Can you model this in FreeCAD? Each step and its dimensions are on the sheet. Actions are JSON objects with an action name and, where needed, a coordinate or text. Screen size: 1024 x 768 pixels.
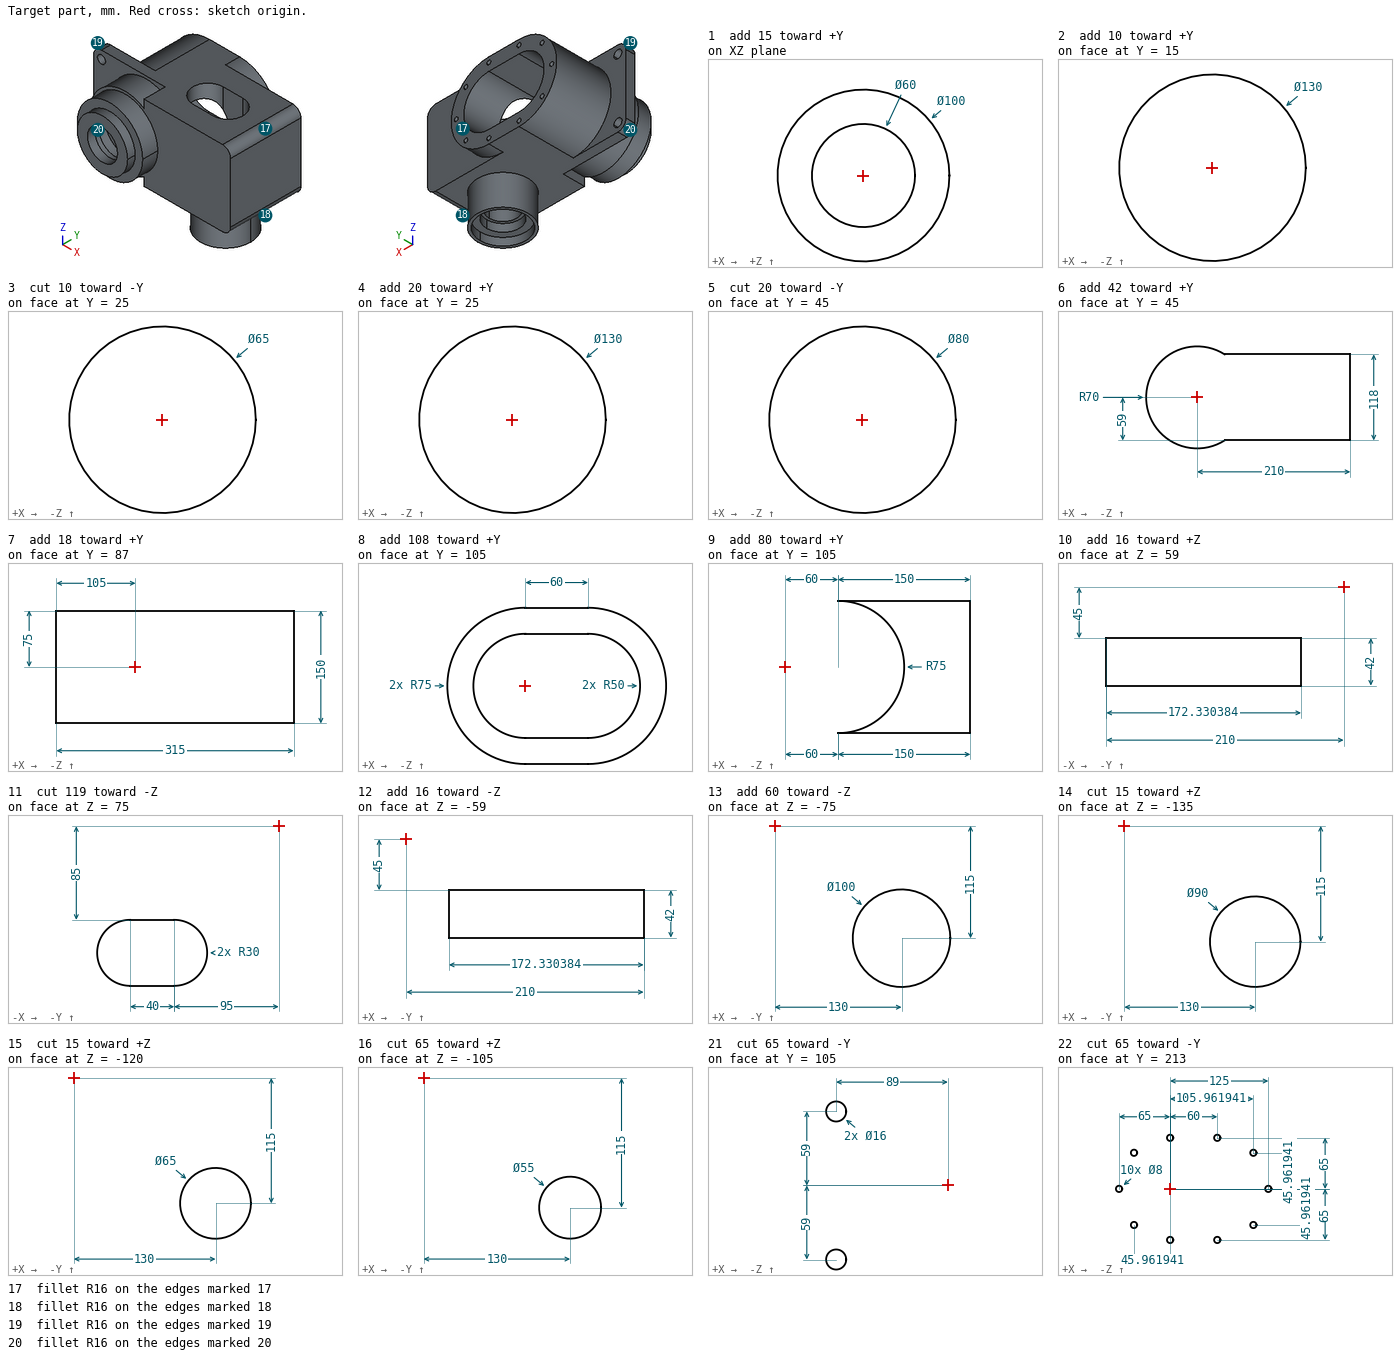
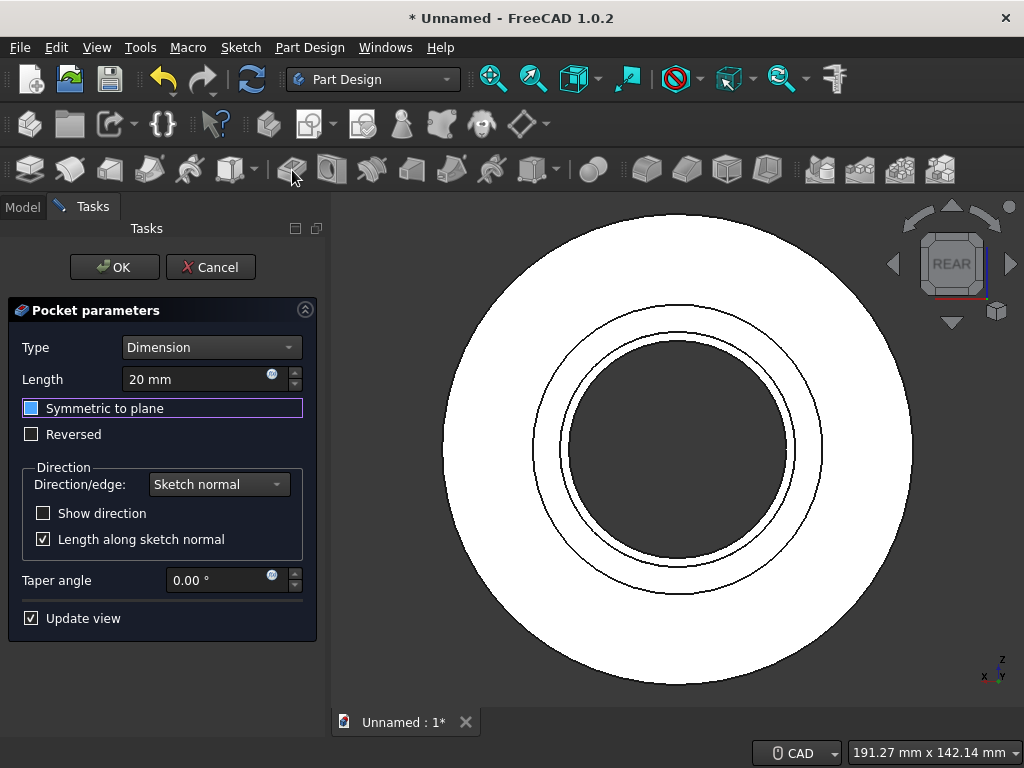
{"action": "left_click", "coordinate": [115, 267]}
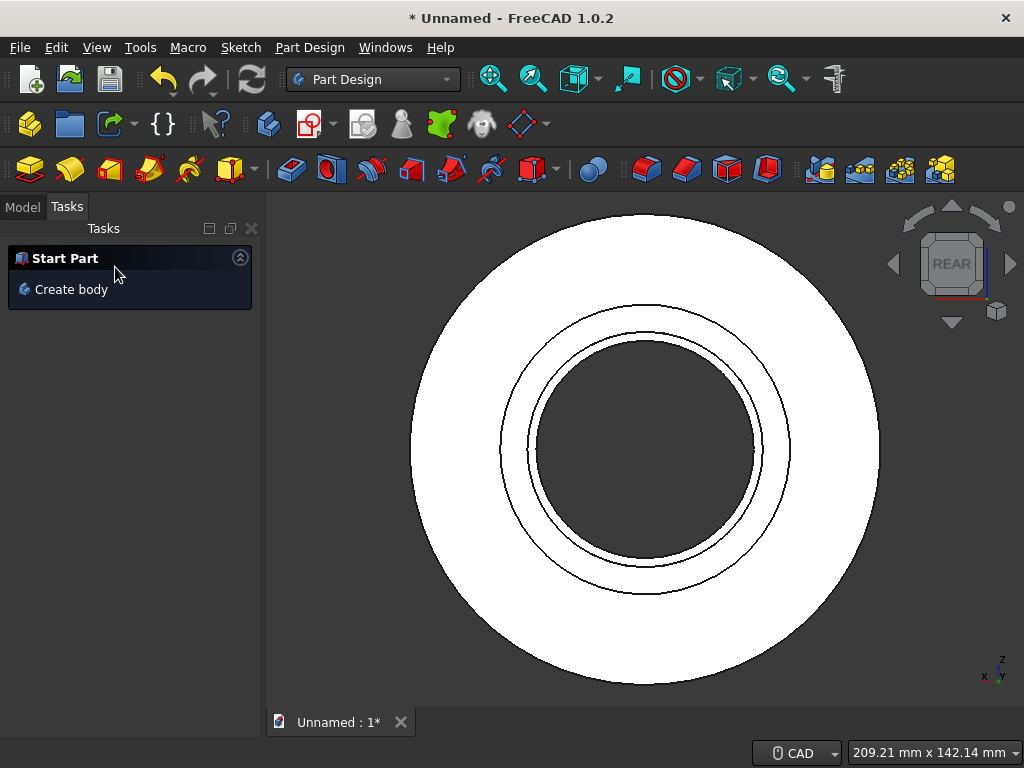
{"action": "left_click", "coordinate": [511, 583]}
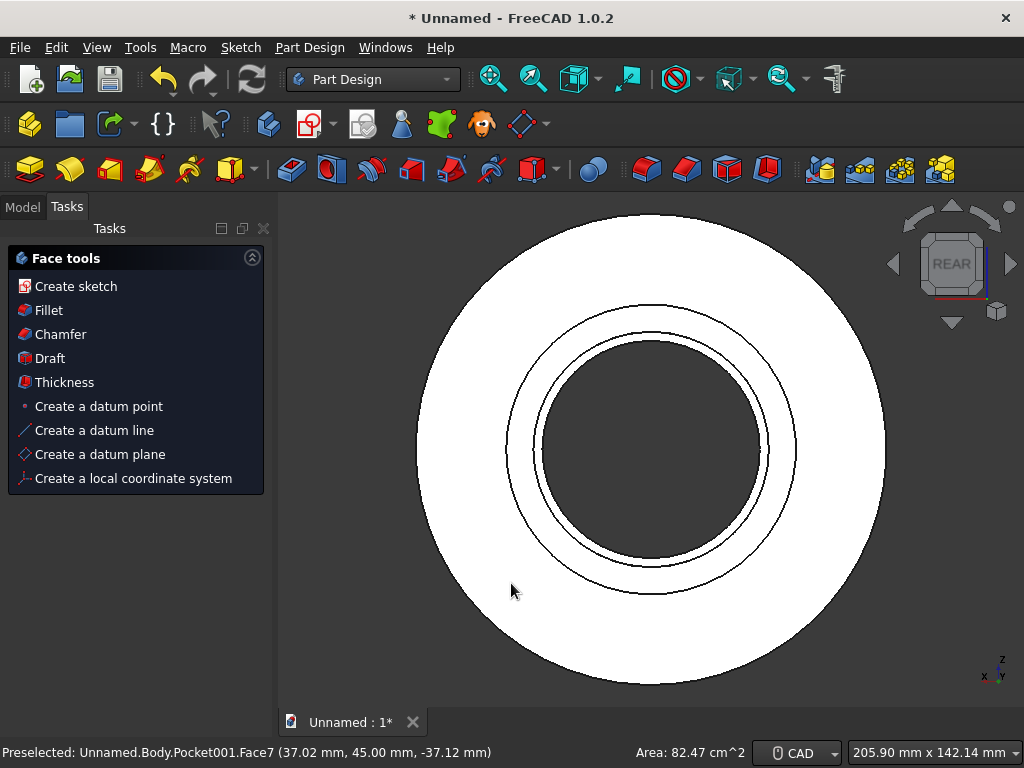
{"action": "left_click", "coordinate": [310, 124]}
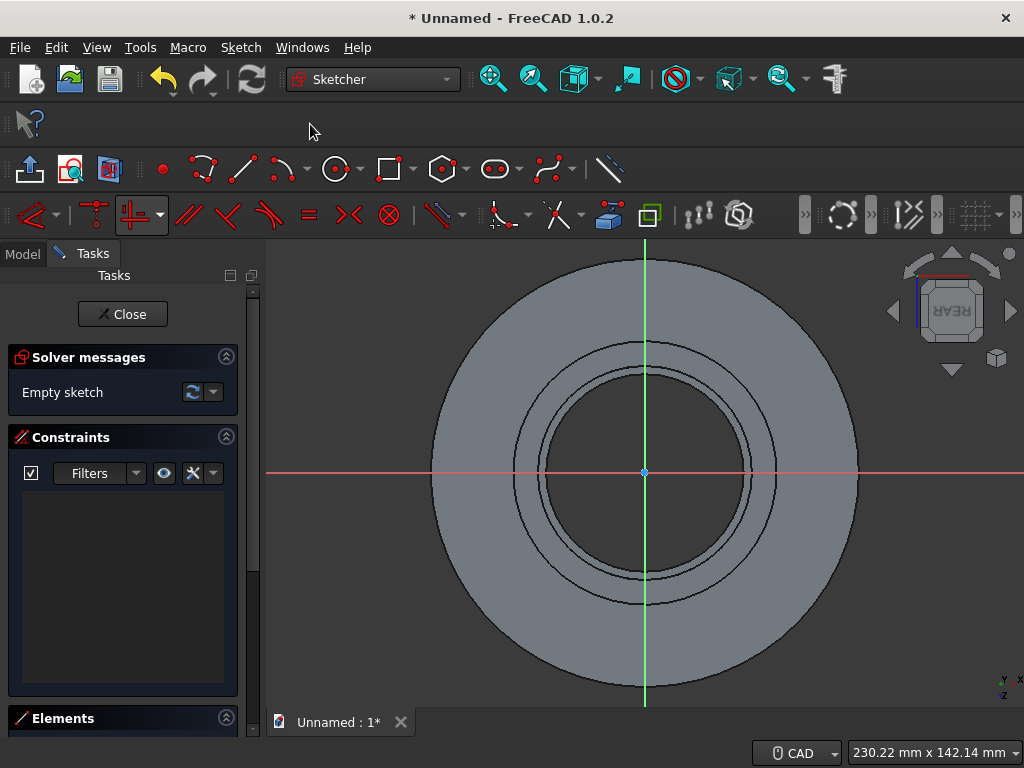
{"action": "scroll", "coordinate": [333, 473], "scroll_direction": "down", "scroll_amount": 4}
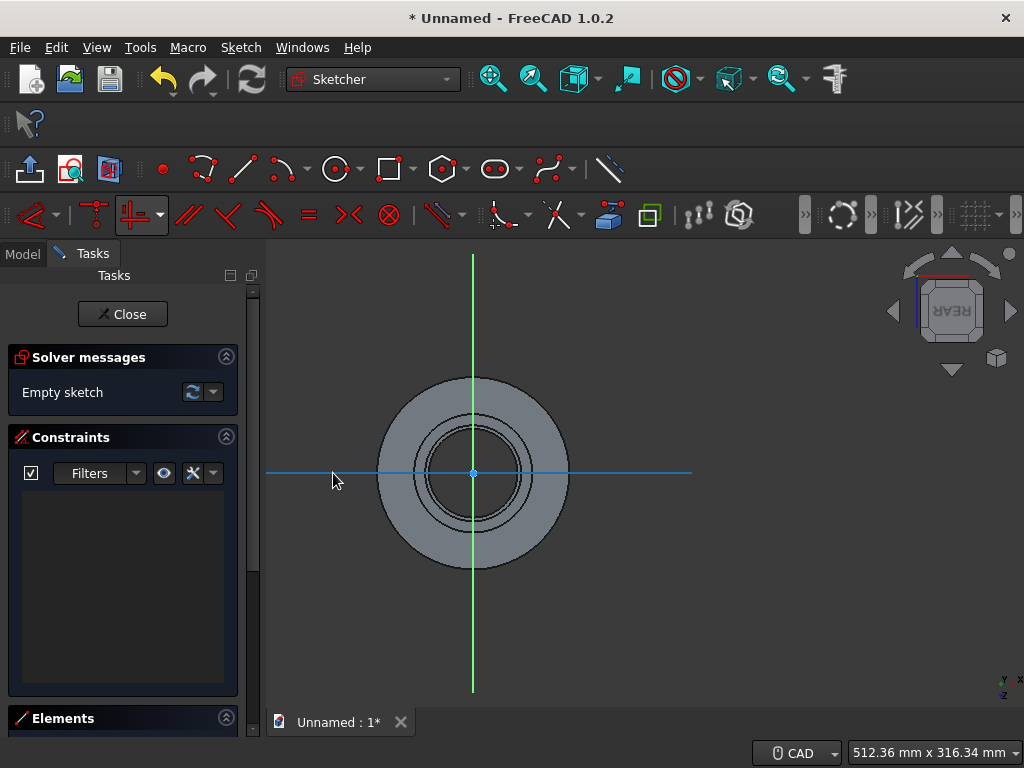
{"action": "left_click", "coordinate": [204, 170]}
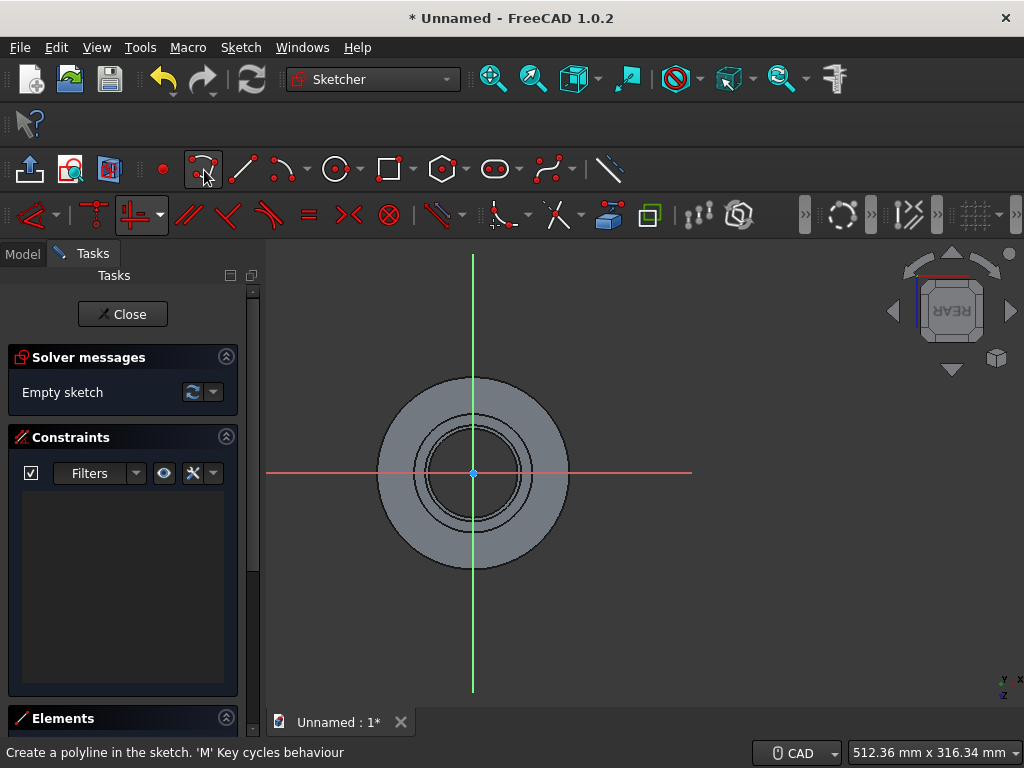
{"action": "left_click", "coordinate": [529, 561]}
{"action": "left_click", "coordinate": [784, 561]}
{"action": "left_click", "coordinate": [784, 386]}
{"action": "left_click", "coordinate": [529, 386]}
{"action": "right_click", "coordinate": [529, 386]}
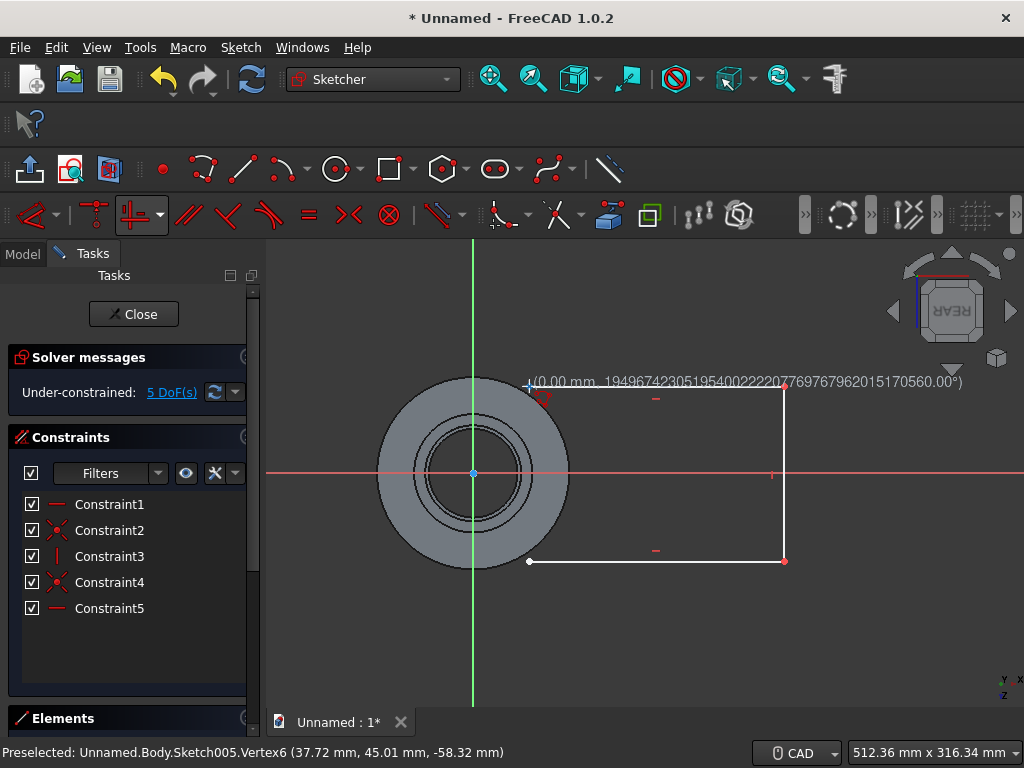
{"action": "key", "text": "g 3 a"}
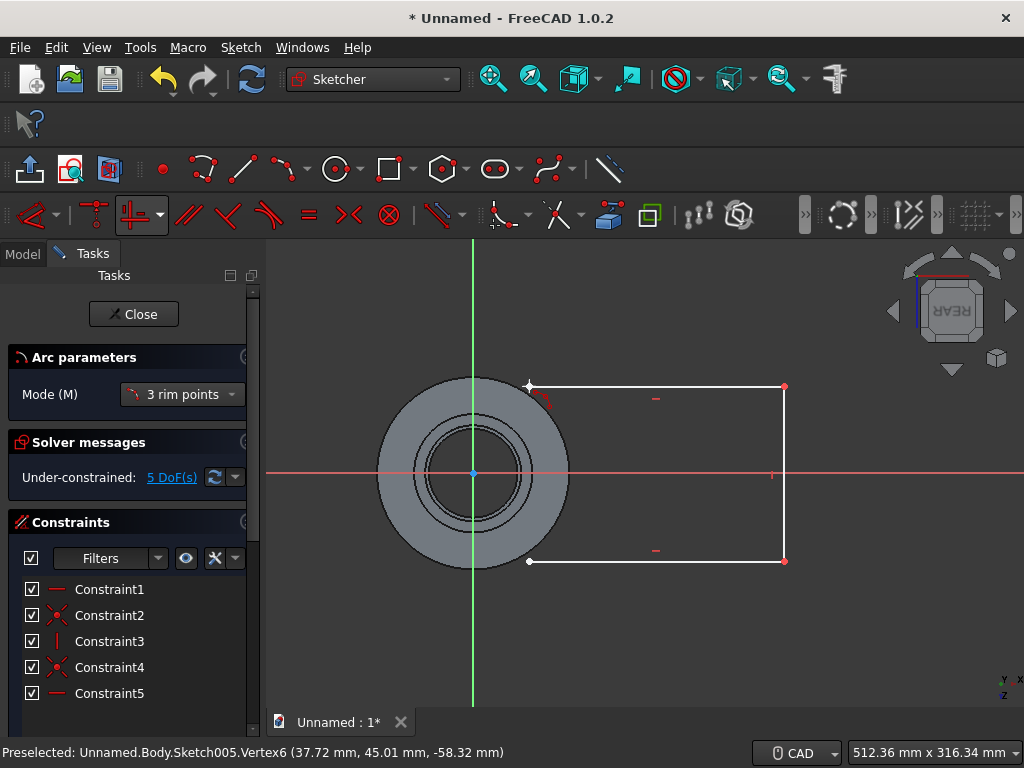
{"action": "left_click", "coordinate": [529, 387]}
{"action": "left_click", "coordinate": [529, 562]}
{"action": "left_click", "coordinate": [379, 430]}
{"action": "key", "text": "Escape"}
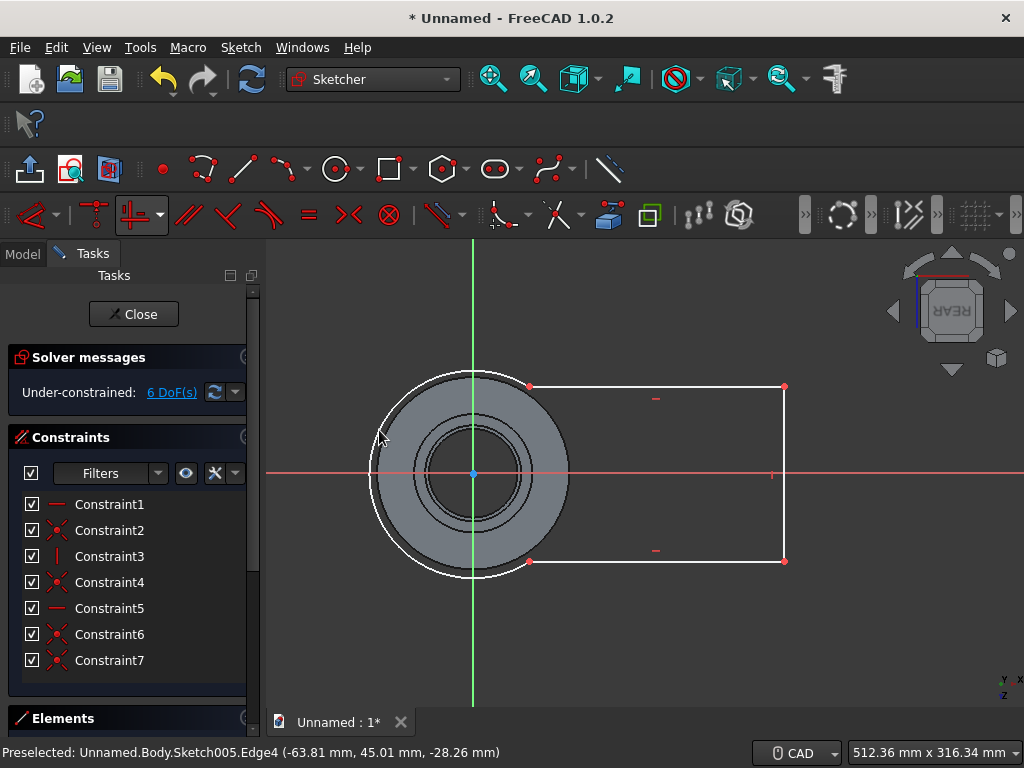
{"action": "left_click_drag", "start_coordinate": [463, 463], "coordinate": [483, 484]}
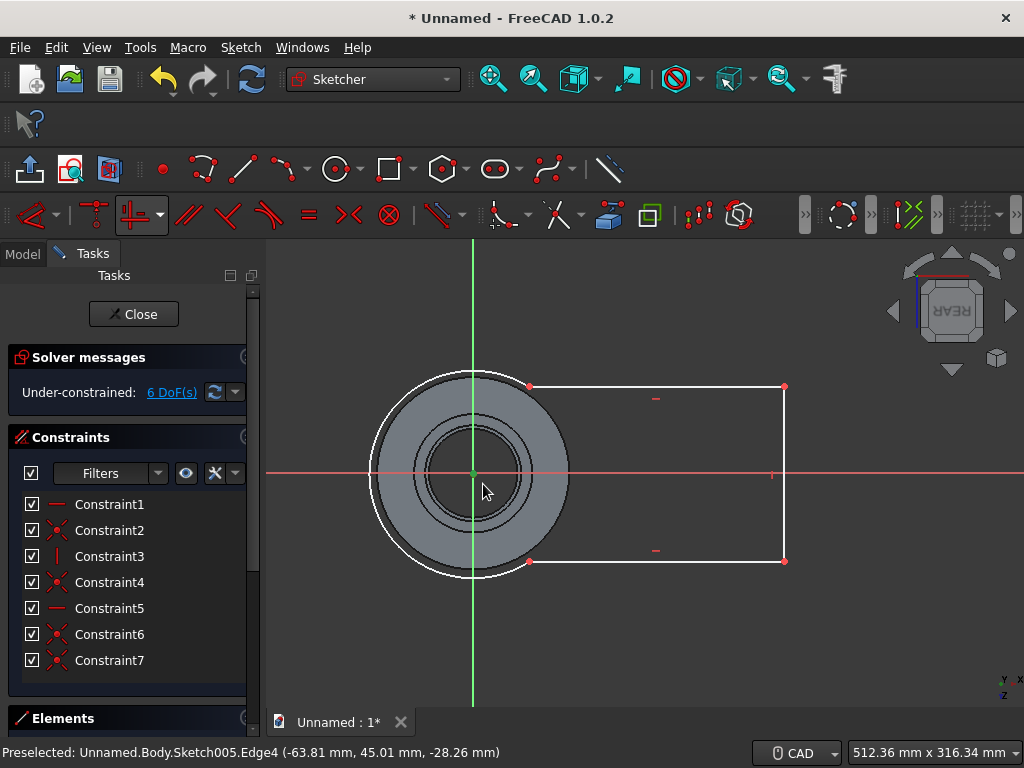
{"action": "left_click", "coordinate": [94, 216]}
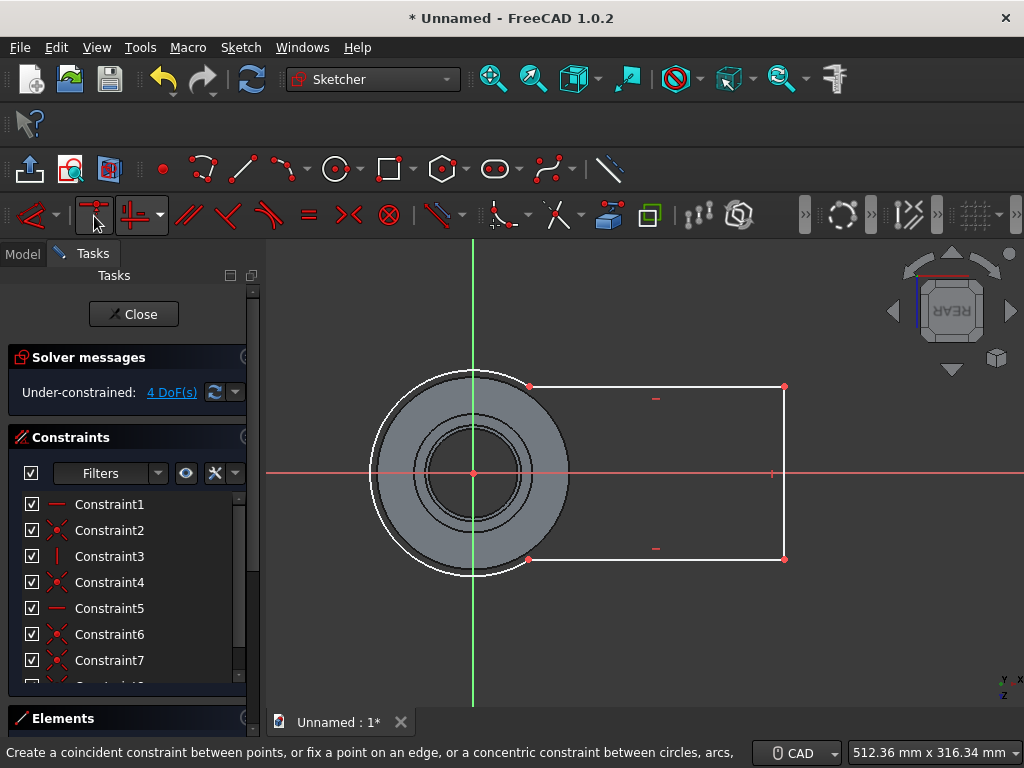
{"action": "left_click", "coordinate": [32, 216]}